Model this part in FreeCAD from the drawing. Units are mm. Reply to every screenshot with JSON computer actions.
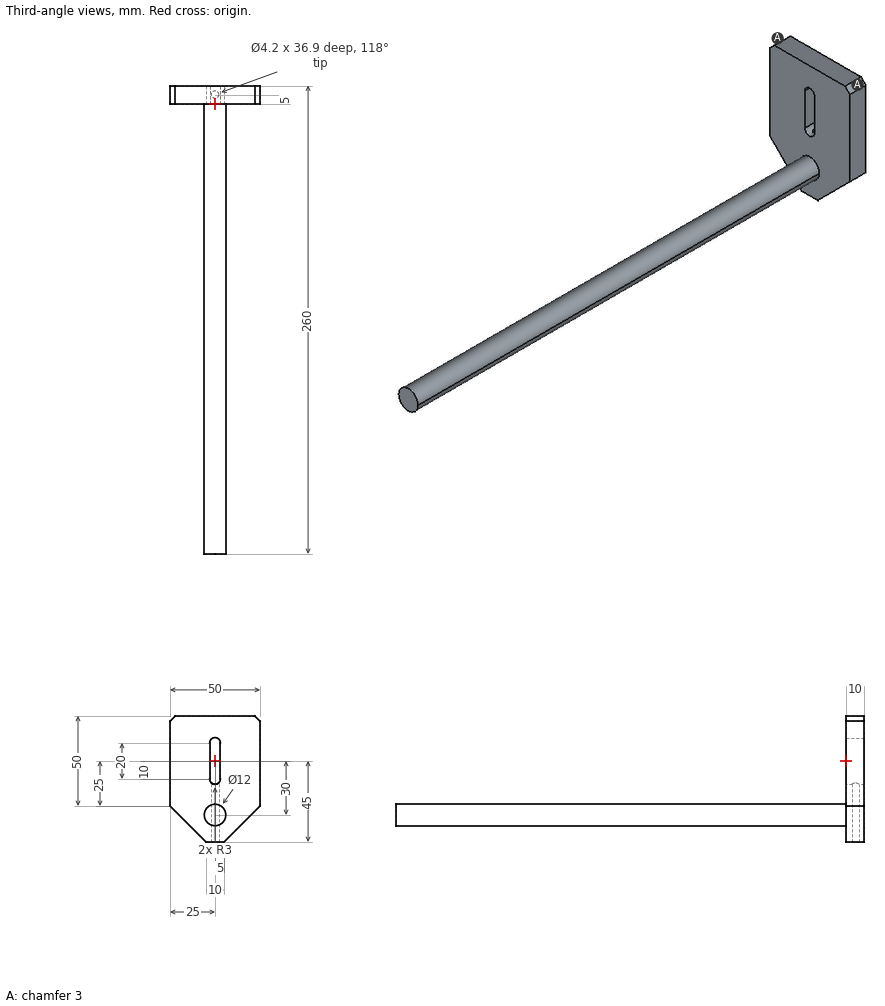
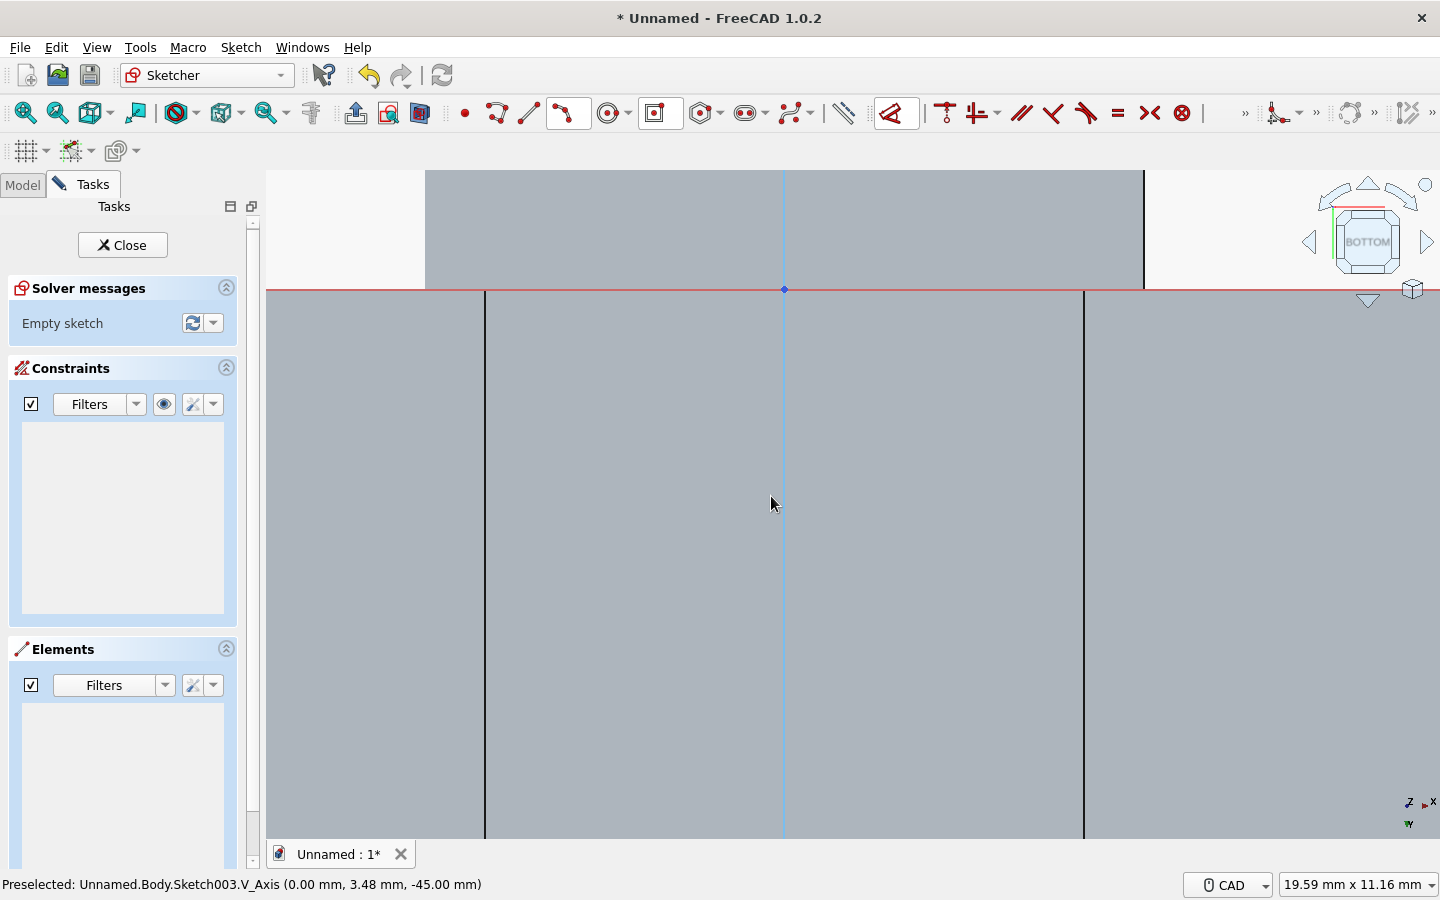
{"action": "left_click", "coordinate": [608, 114]}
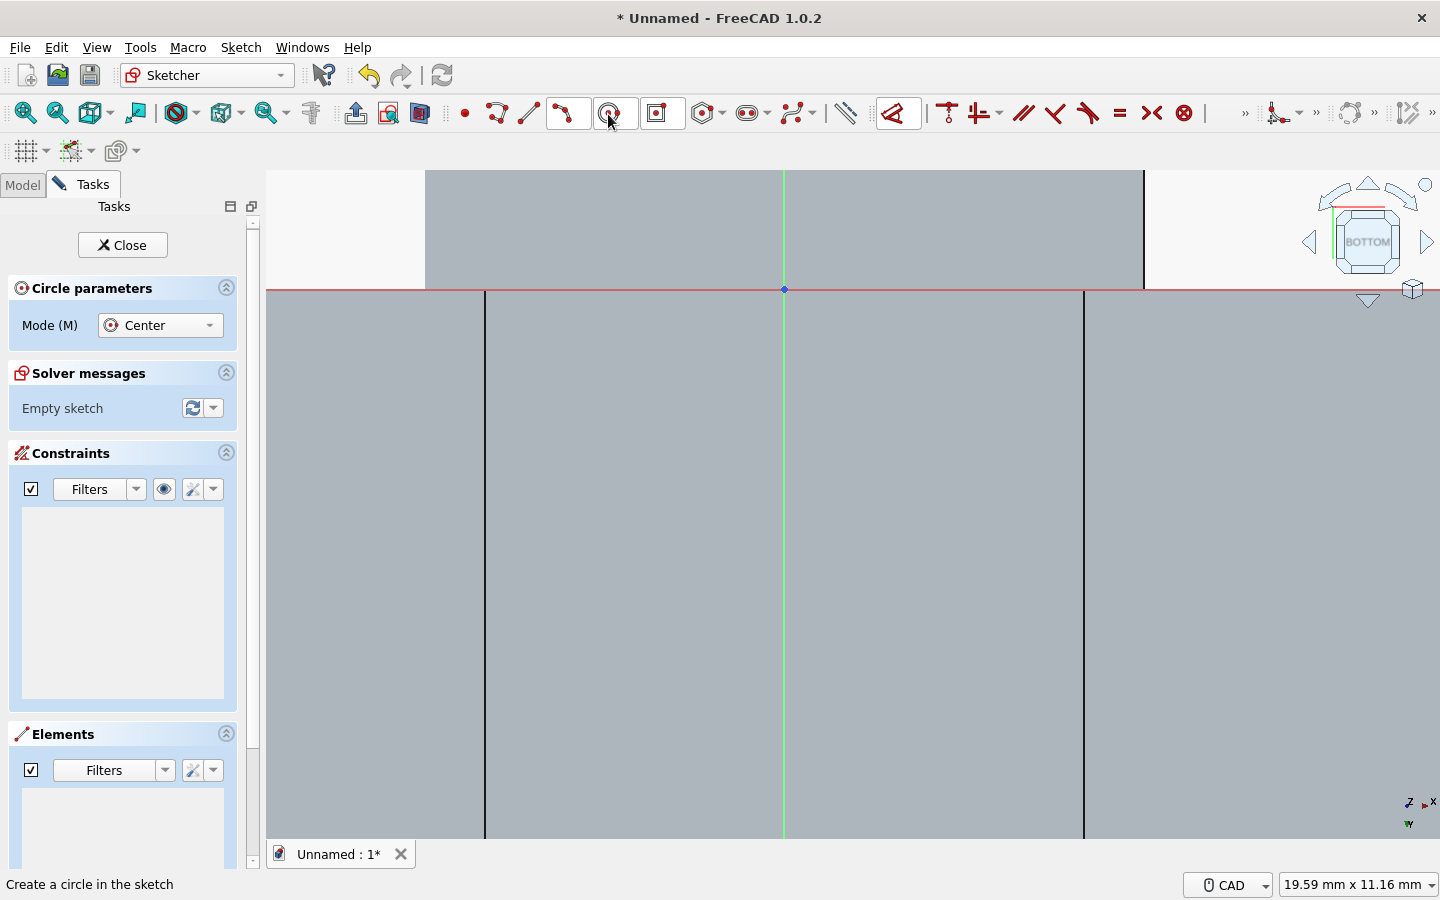
{"action": "left_click", "coordinate": [784, 589]}
{"action": "mouse_move", "coordinate": [873, 500]}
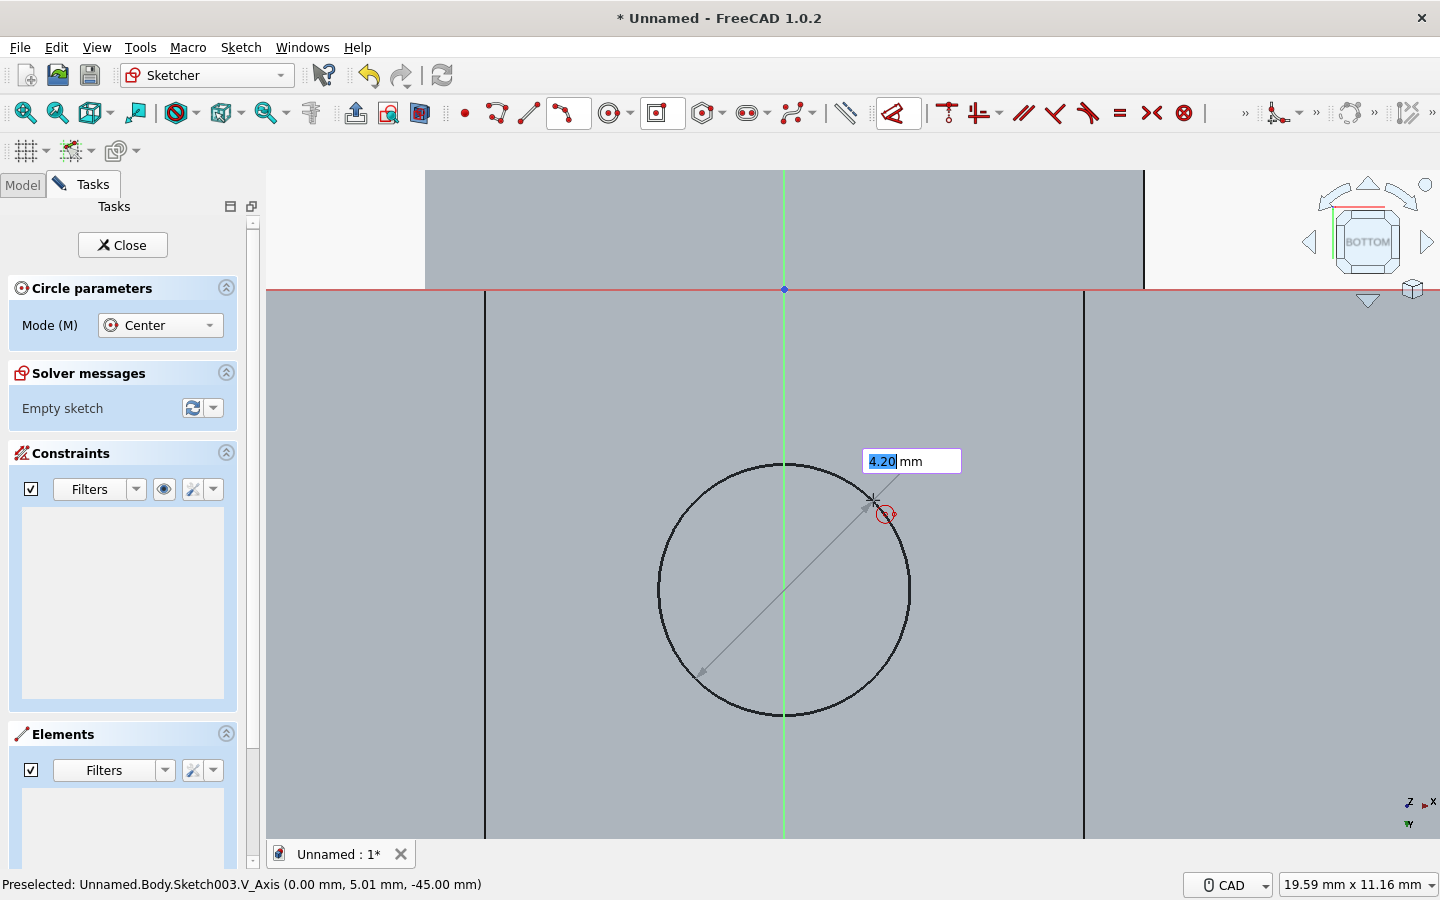
{"action": "type", "text": "4.2"}
{"action": "key", "text": "Return"}
{"action": "key", "text": "Escape"}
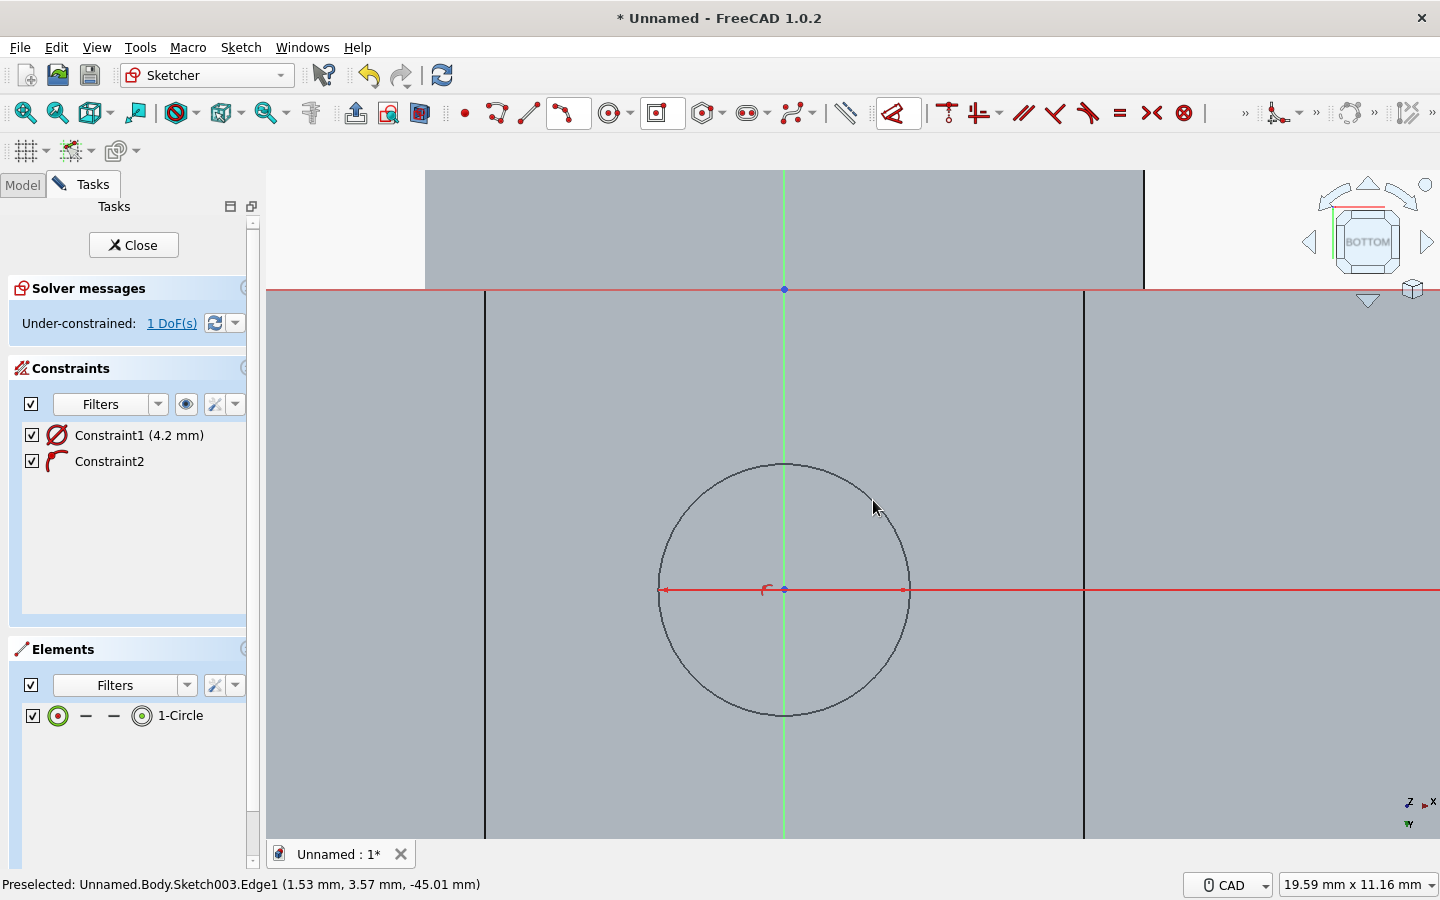
{"action": "left_click", "coordinate": [784, 590]}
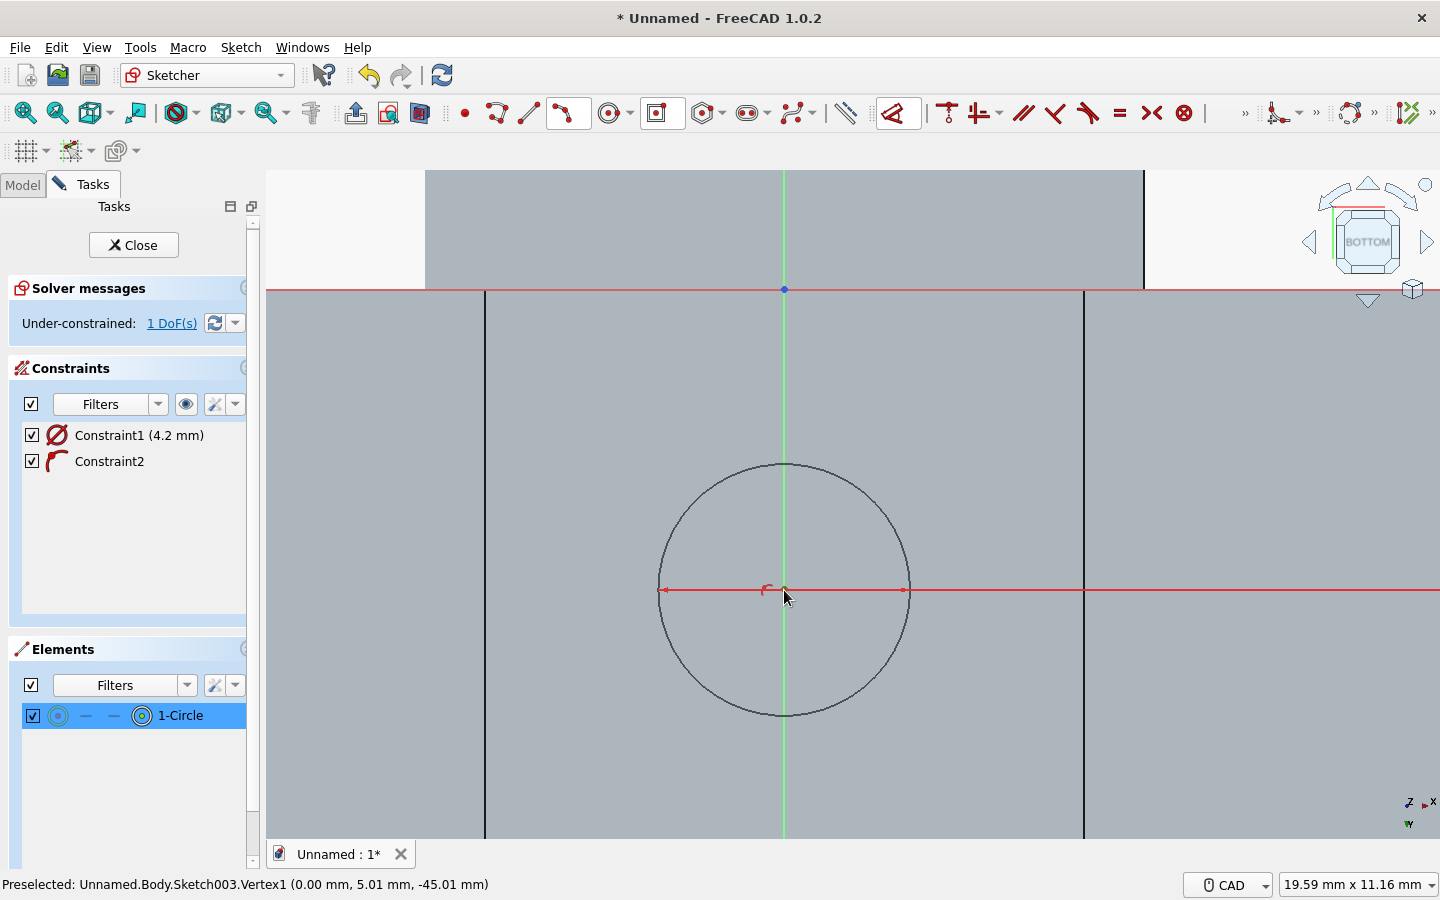
{"action": "key", "text": "i"}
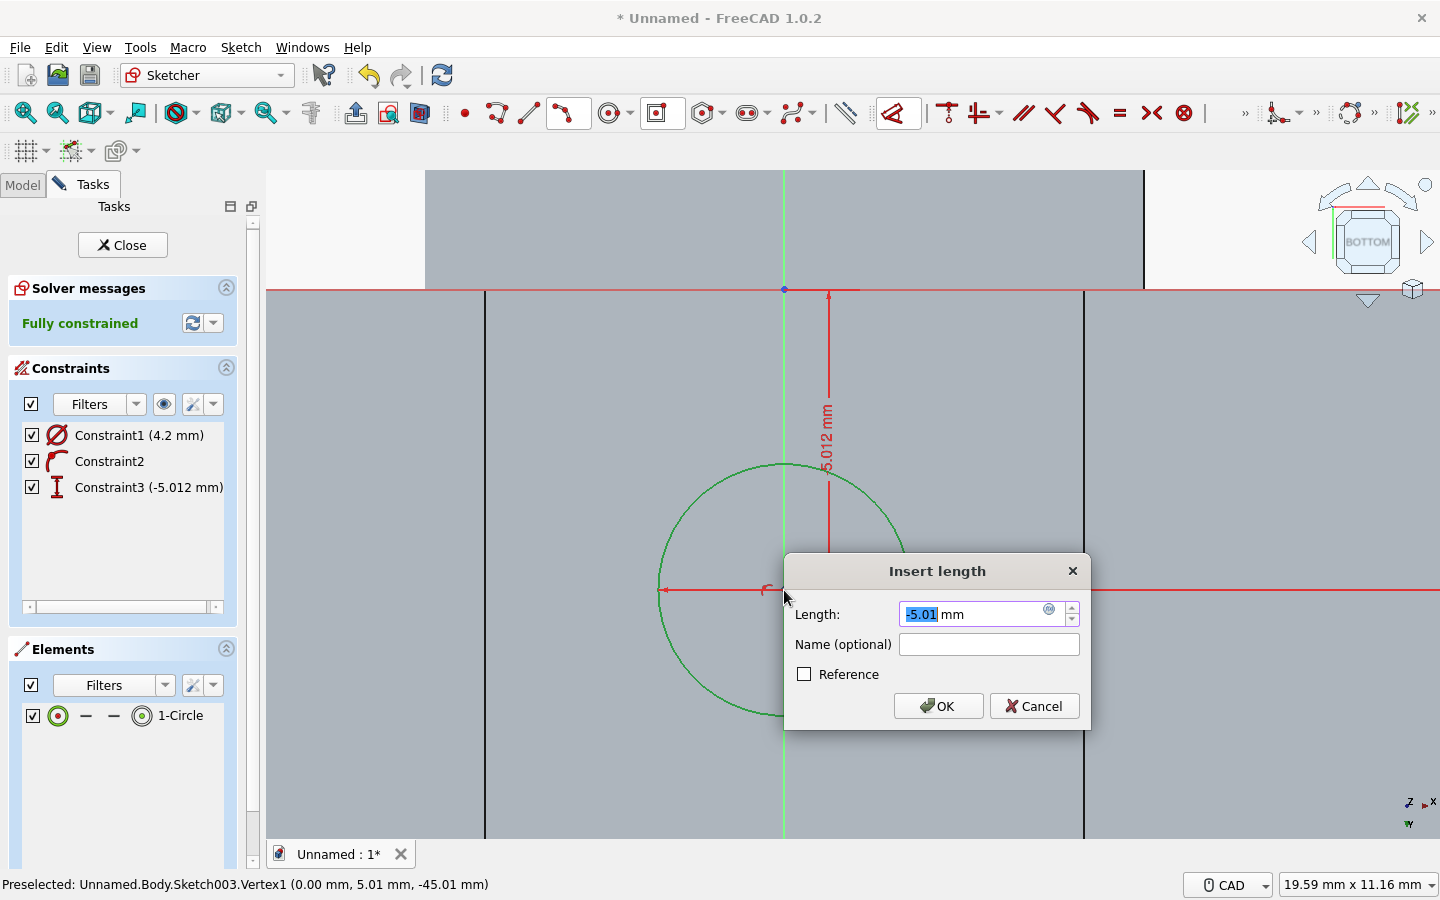
{"action": "type", "text": "-5"}
{"action": "key", "text": "Return"}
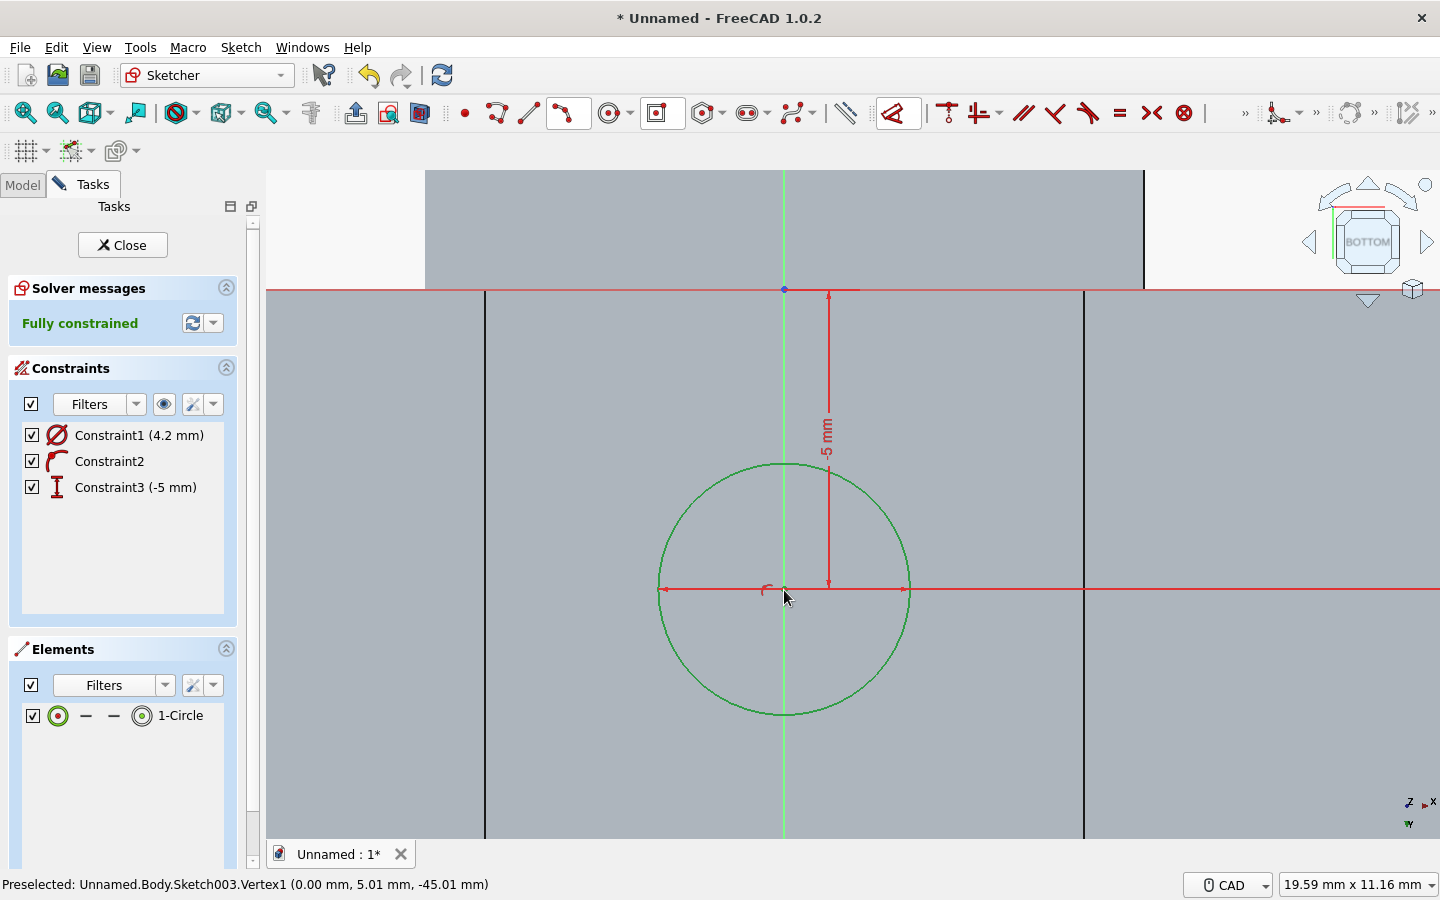
{"action": "left_click", "coordinate": [123, 245]}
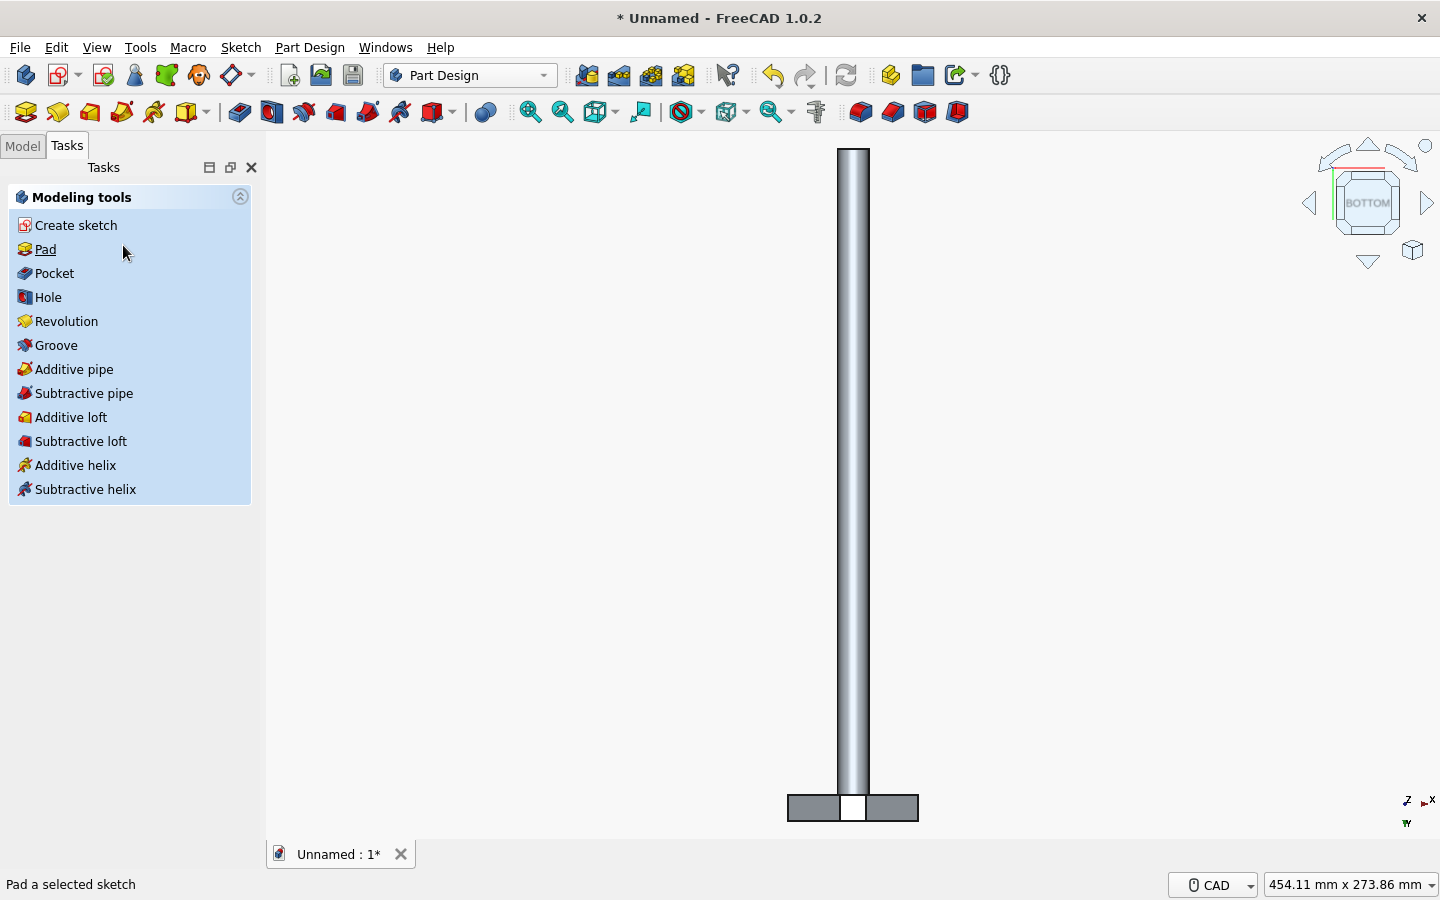
{"action": "left_click", "coordinate": [272, 112]}